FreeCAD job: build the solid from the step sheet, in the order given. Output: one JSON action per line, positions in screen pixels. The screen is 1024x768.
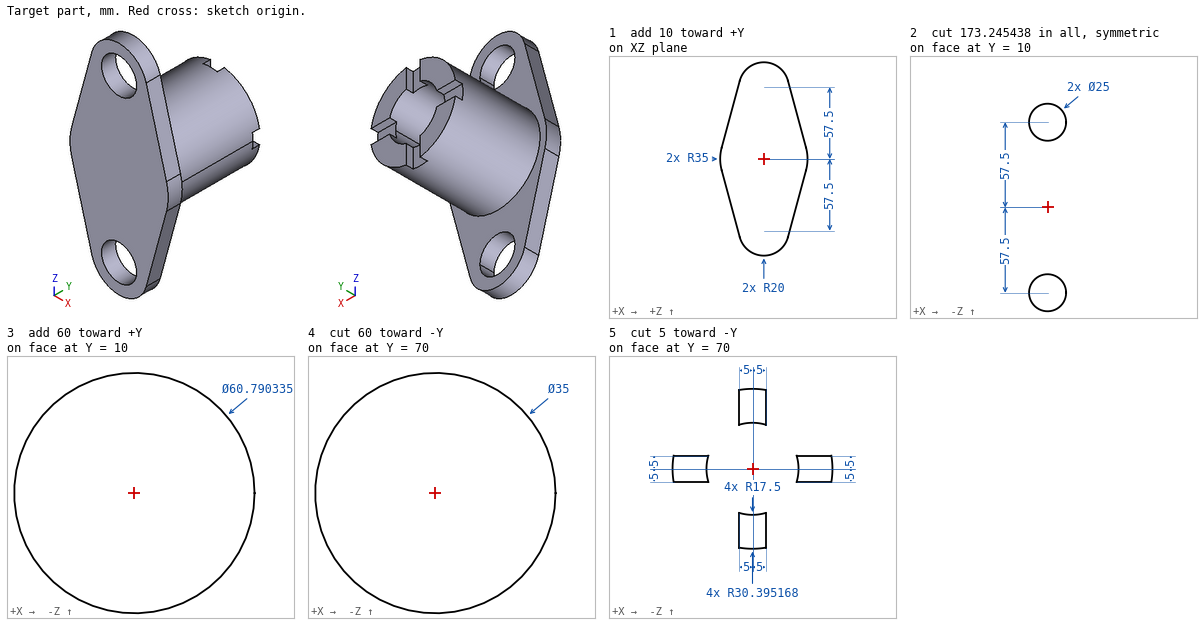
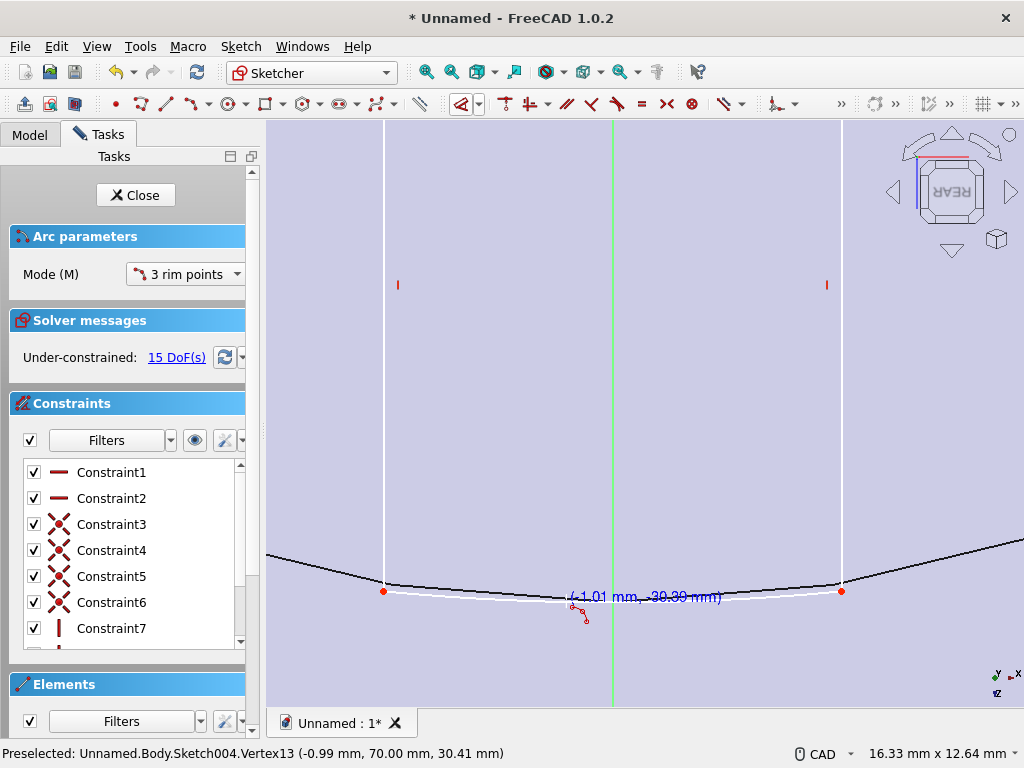
{"action": "scroll", "coordinate": [571, 605], "scroll_direction": "down", "scroll_amount": 10}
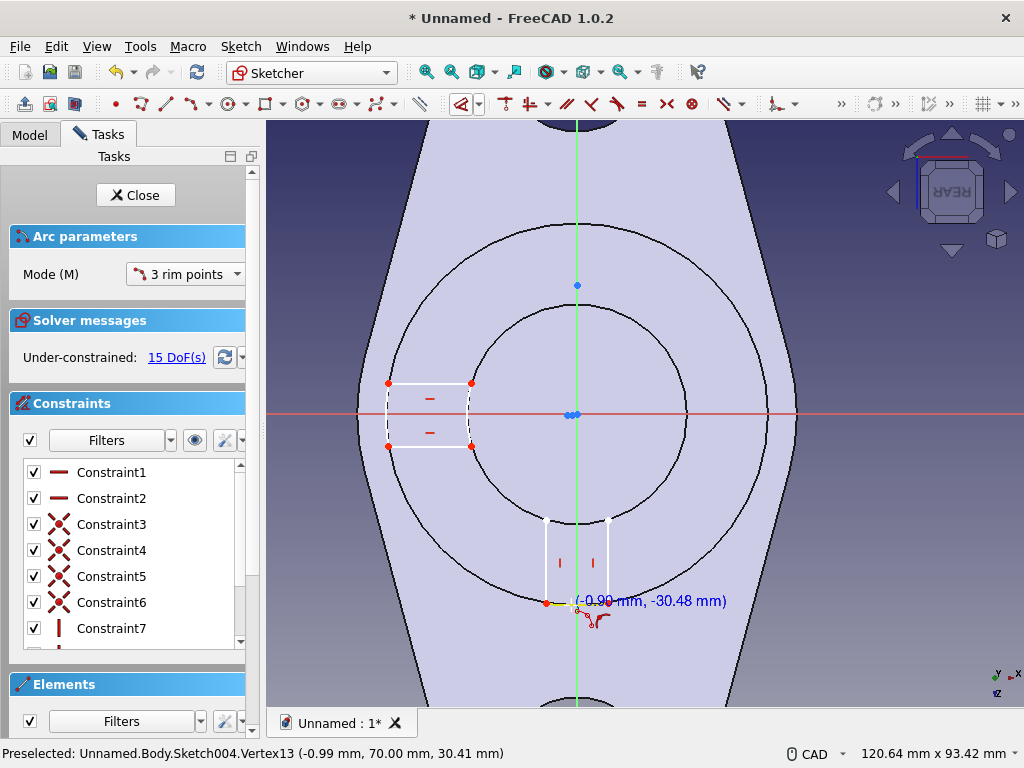
{"action": "left_click", "coordinate": [608, 521]}
{"action": "left_click", "coordinate": [546, 521]}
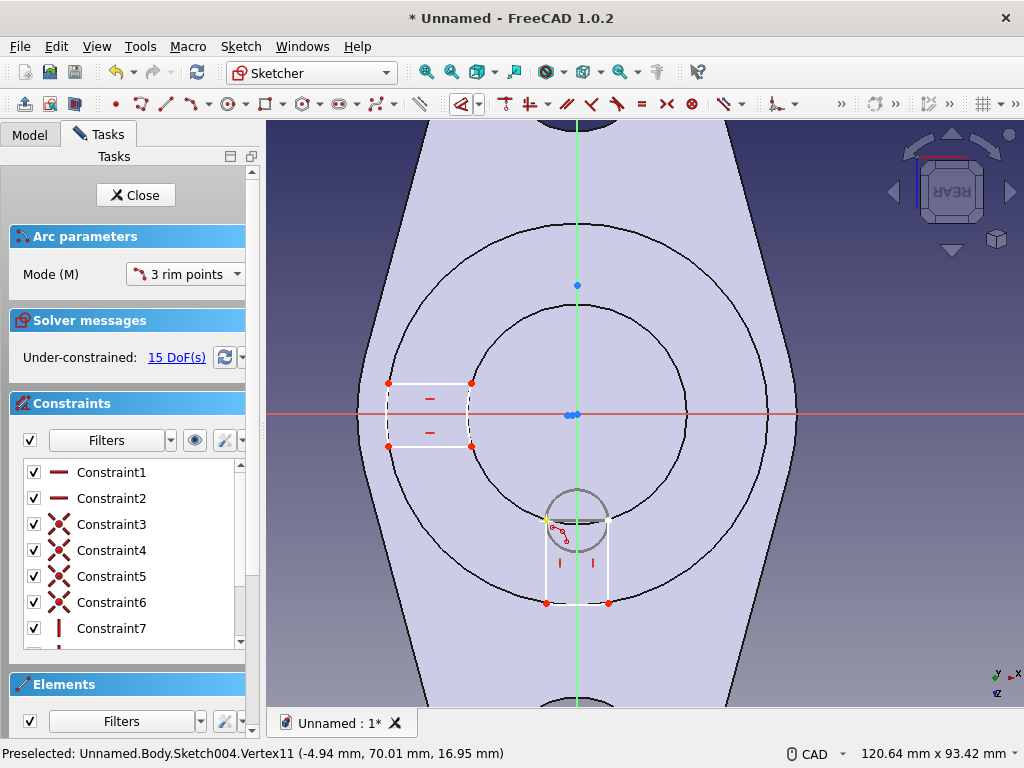
{"action": "scroll", "coordinate": [571, 524], "scroll_direction": "up", "scroll_amount": 7}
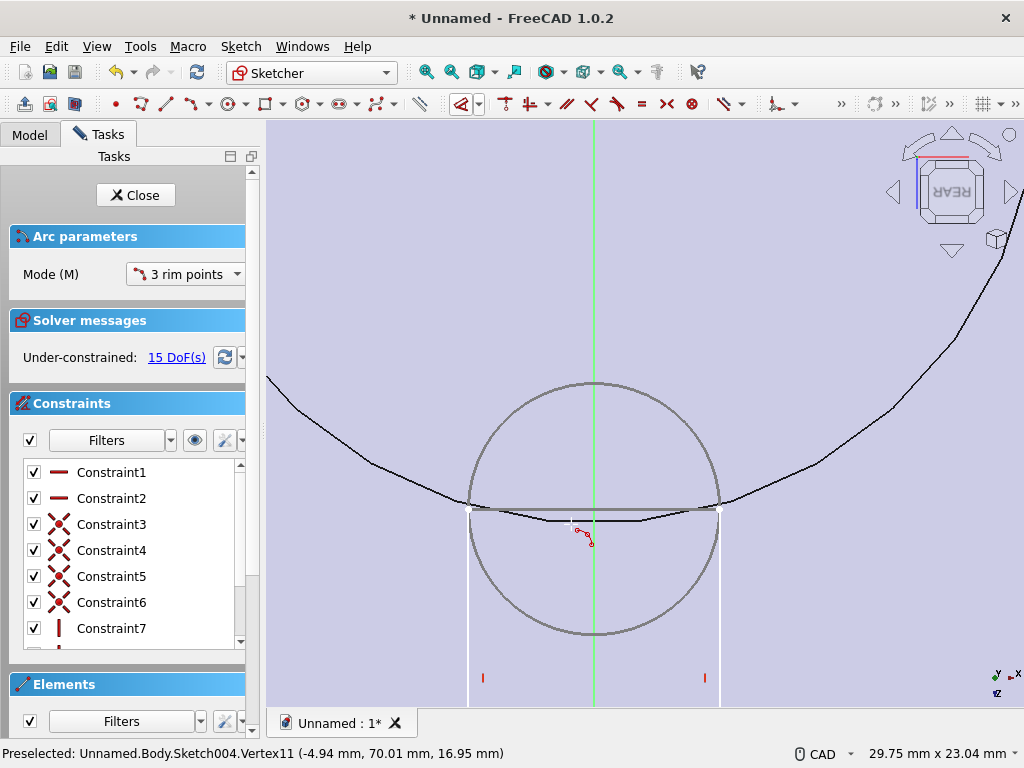
{"action": "left_click", "coordinate": [568, 522]}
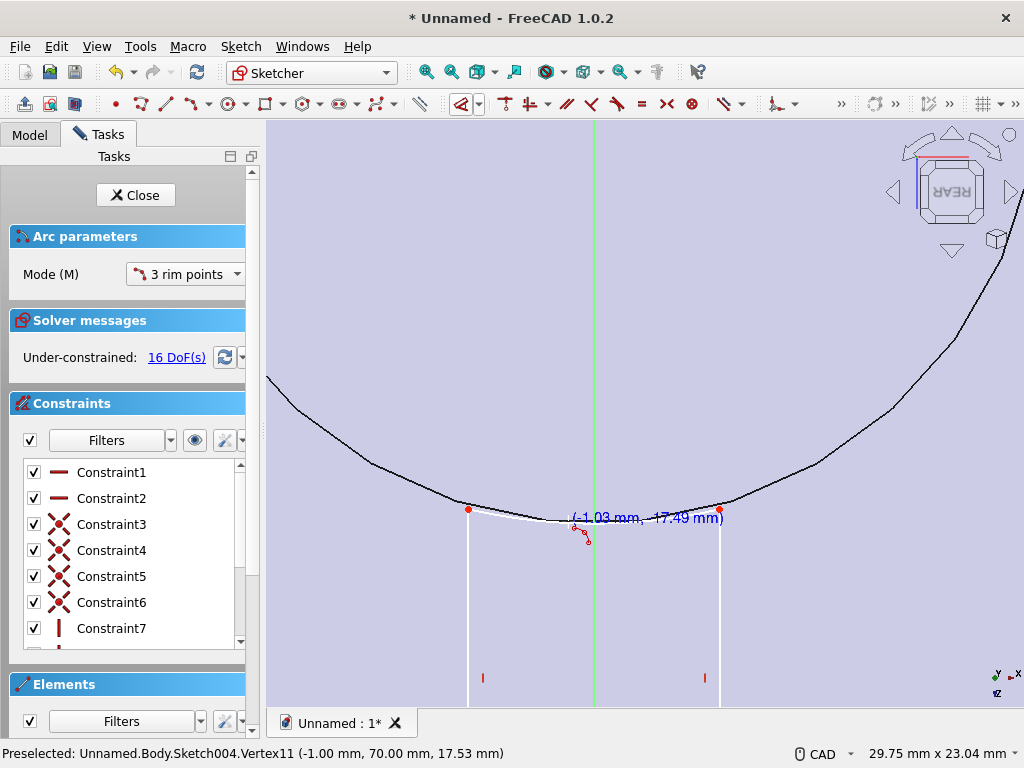
{"action": "left_click", "coordinate": [166, 104]}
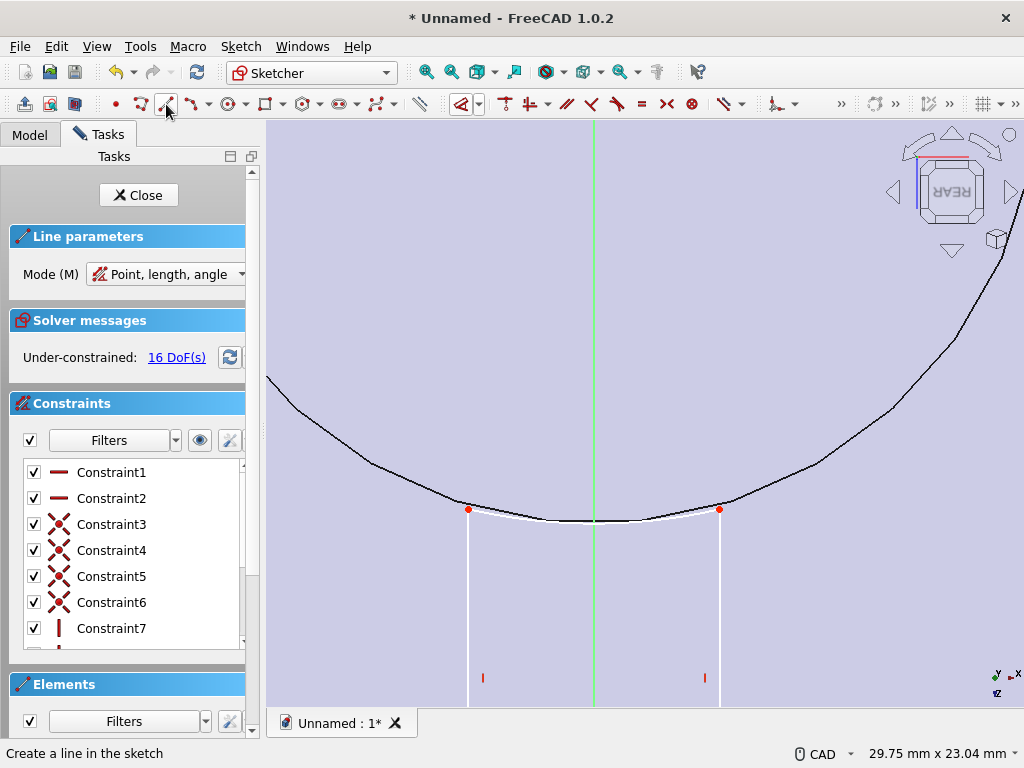
{"action": "scroll", "coordinate": [571, 524], "scroll_direction": "down", "scroll_amount": 7}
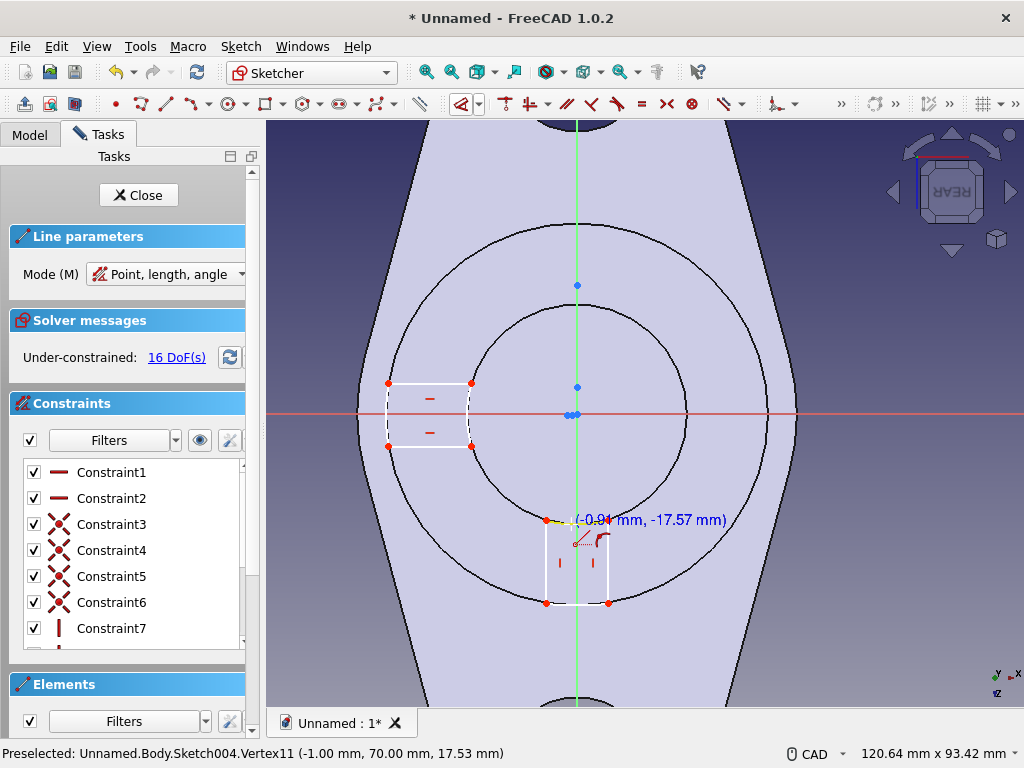
{"action": "left_click", "coordinate": [546, 226]}
{"action": "left_click", "coordinate": [546, 309]}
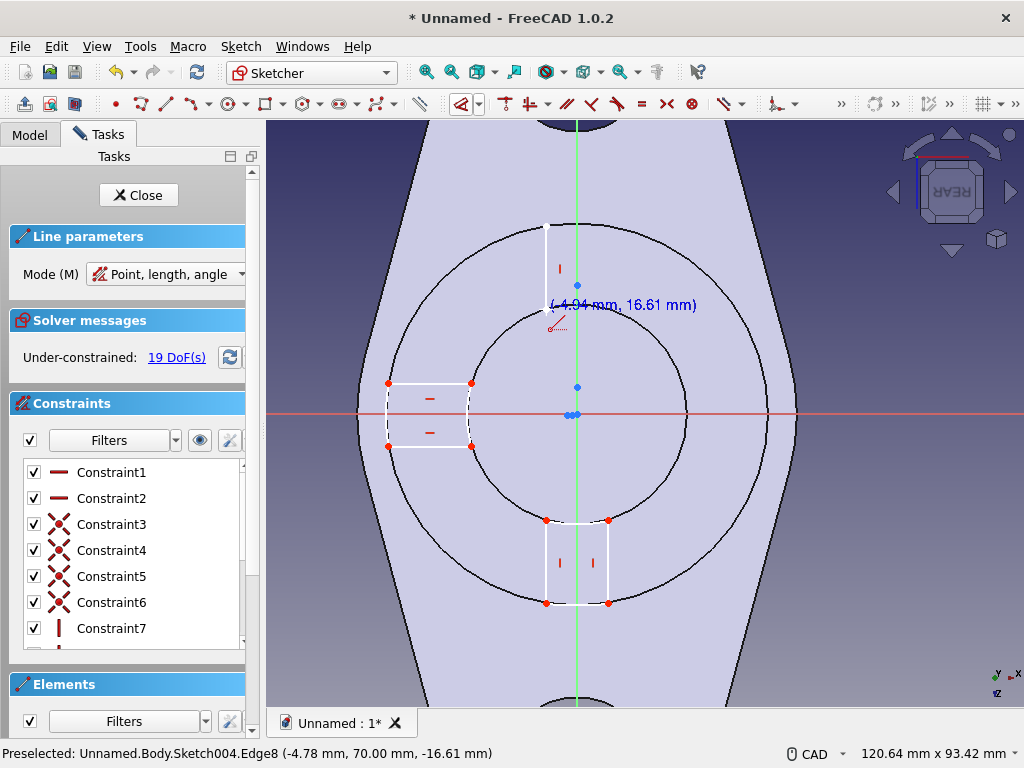
{"action": "left_click", "coordinate": [608, 309]}
{"action": "left_click", "coordinate": [608, 226]}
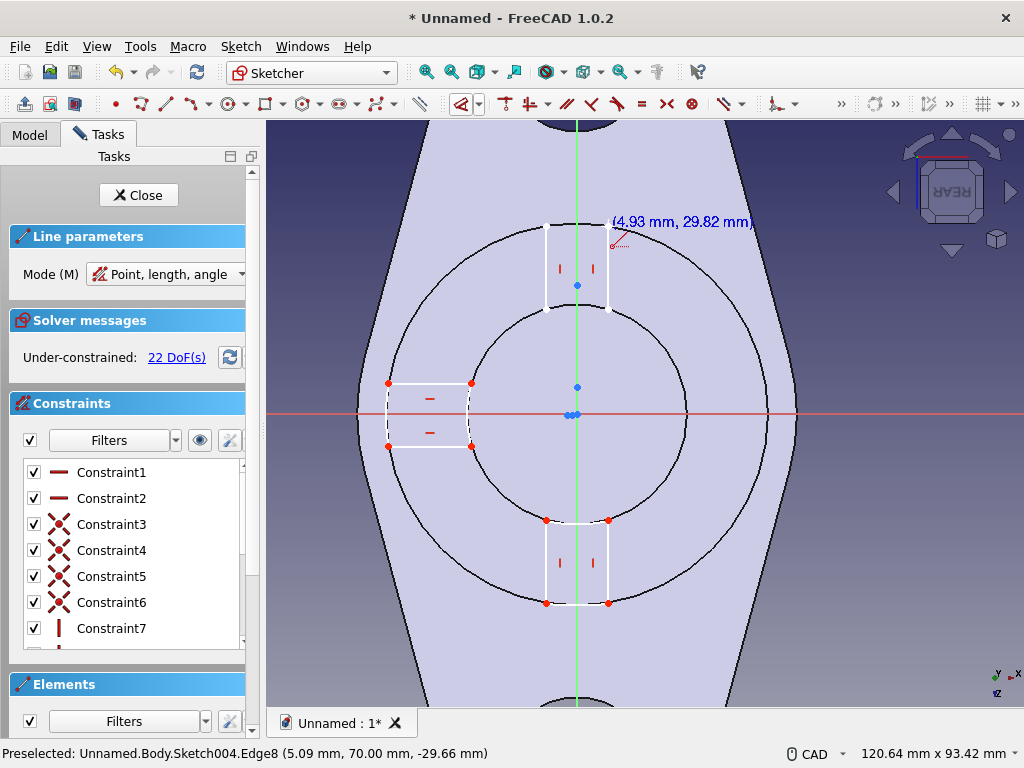
{"action": "left_click", "coordinate": [190, 104]}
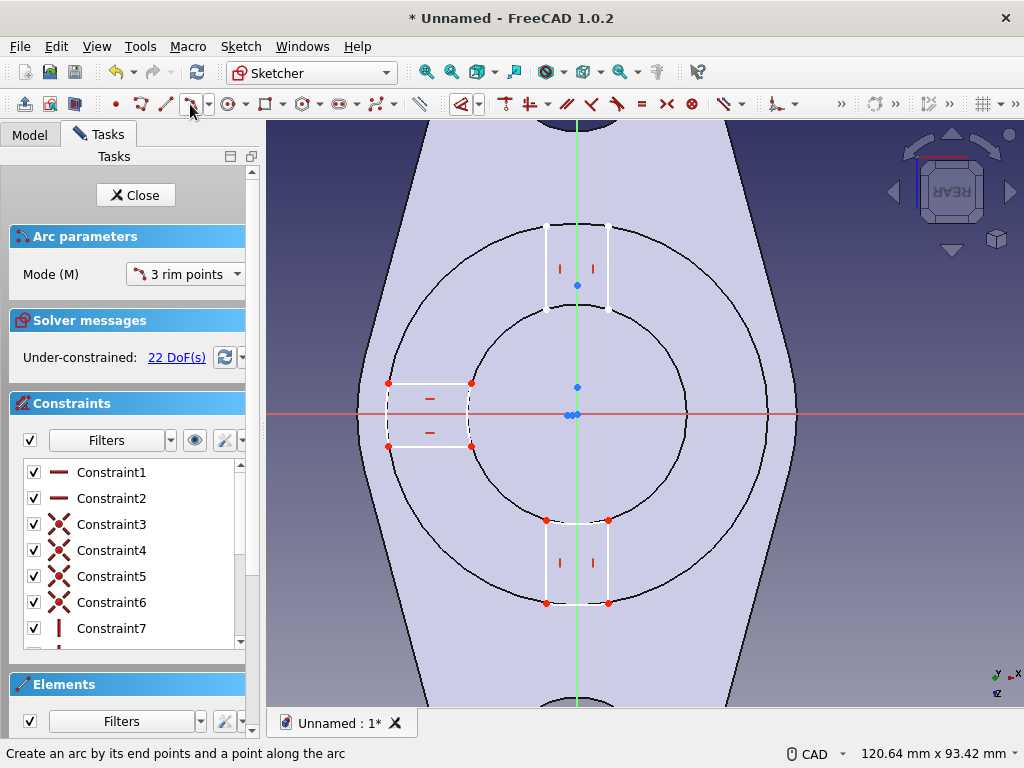
{"action": "left_click", "coordinate": [546, 310]}
{"action": "left_click", "coordinate": [608, 310]}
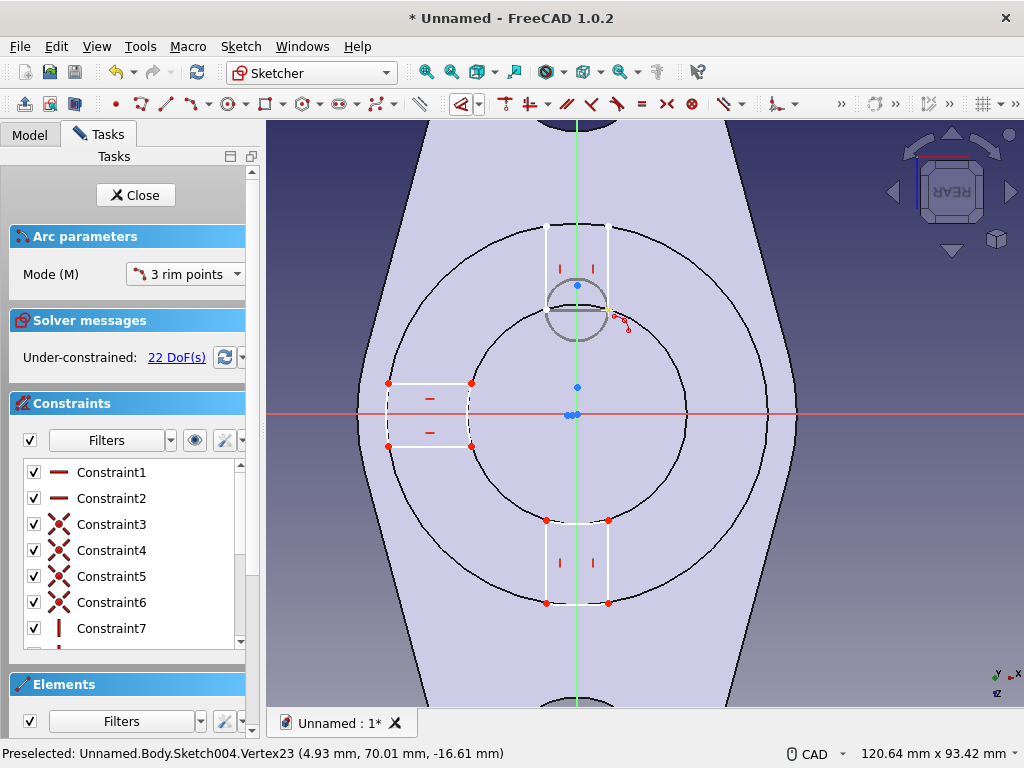
{"action": "scroll", "coordinate": [583, 305], "scroll_direction": "up", "scroll_amount": 7}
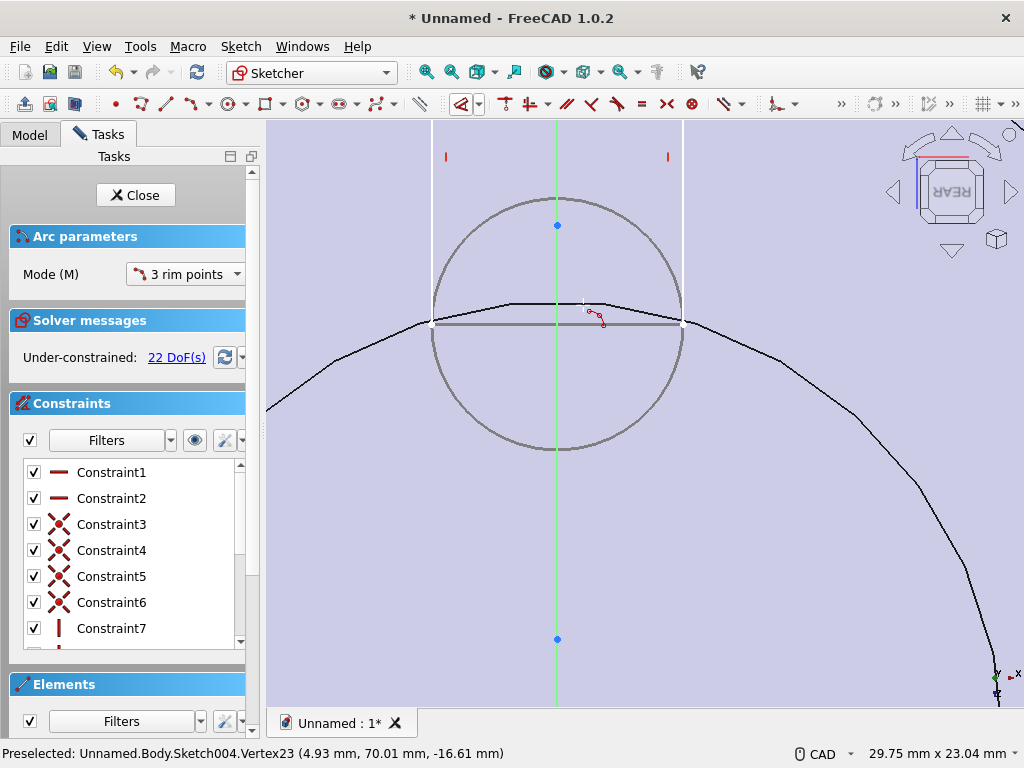
{"action": "left_click", "coordinate": [583, 302]}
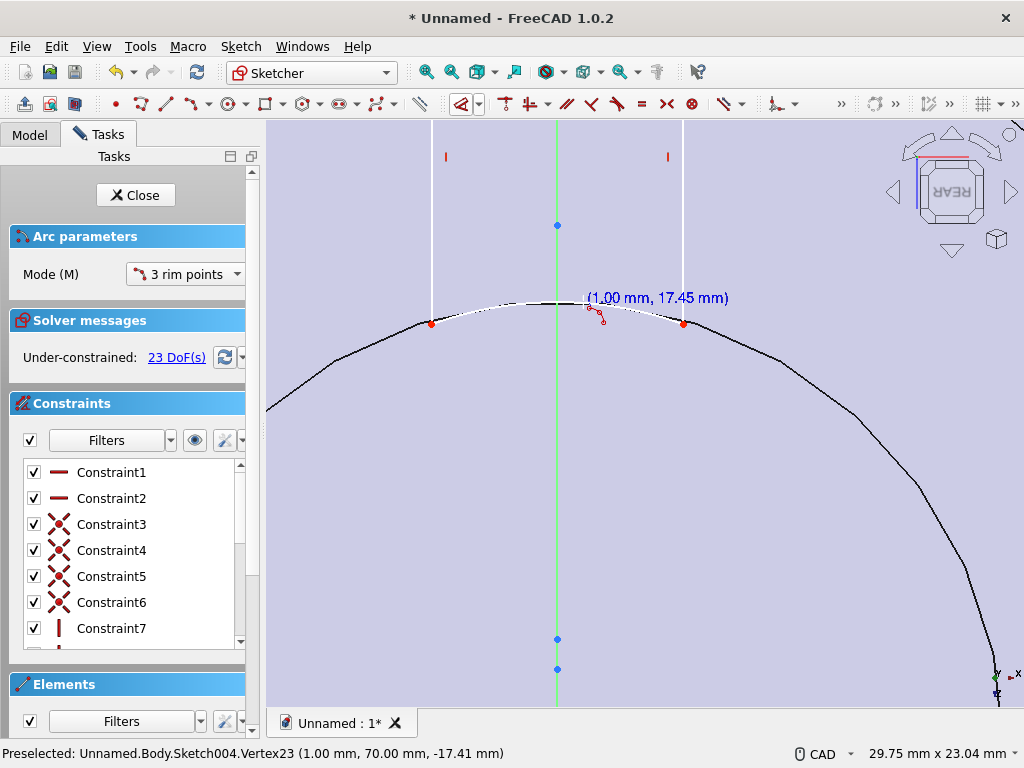
{"action": "scroll", "coordinate": [583, 304], "scroll_direction": "down", "scroll_amount": 7}